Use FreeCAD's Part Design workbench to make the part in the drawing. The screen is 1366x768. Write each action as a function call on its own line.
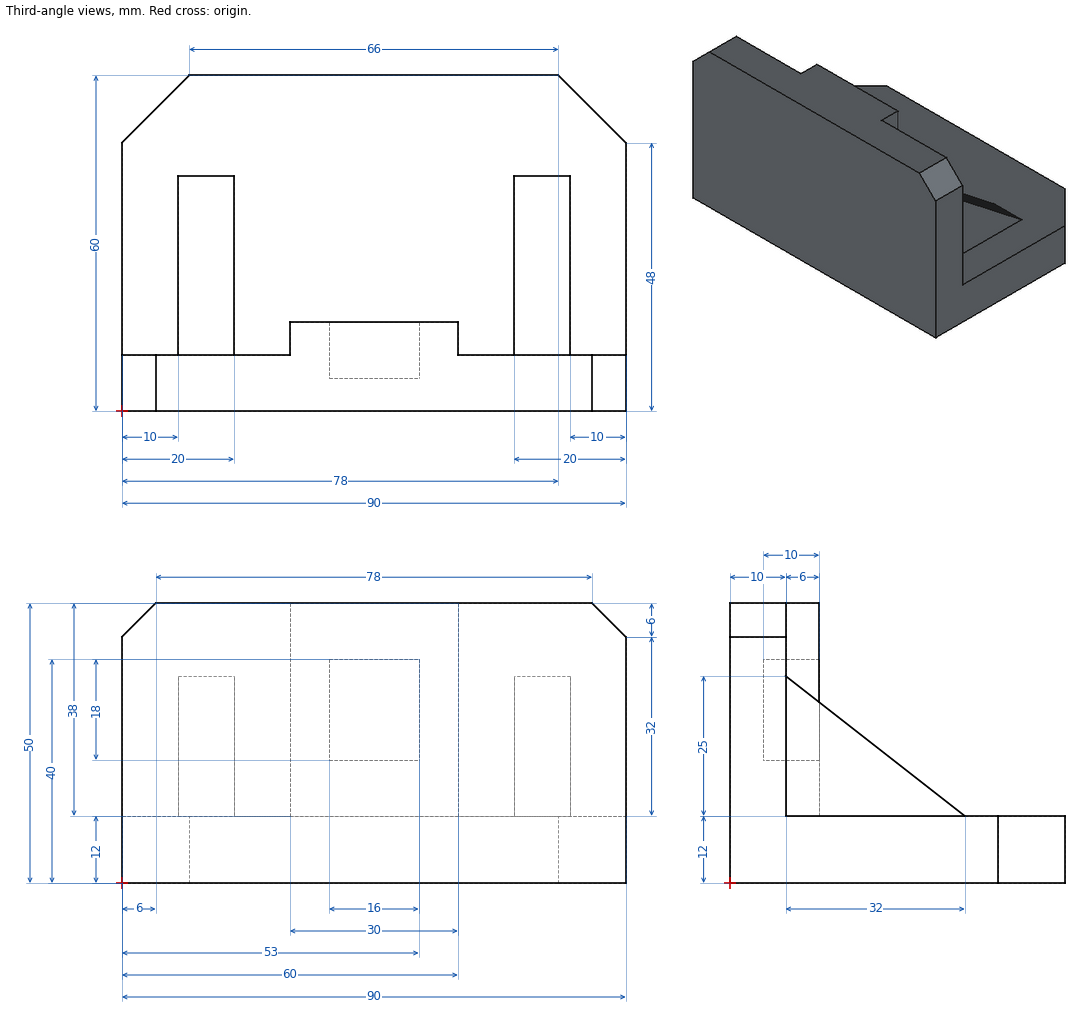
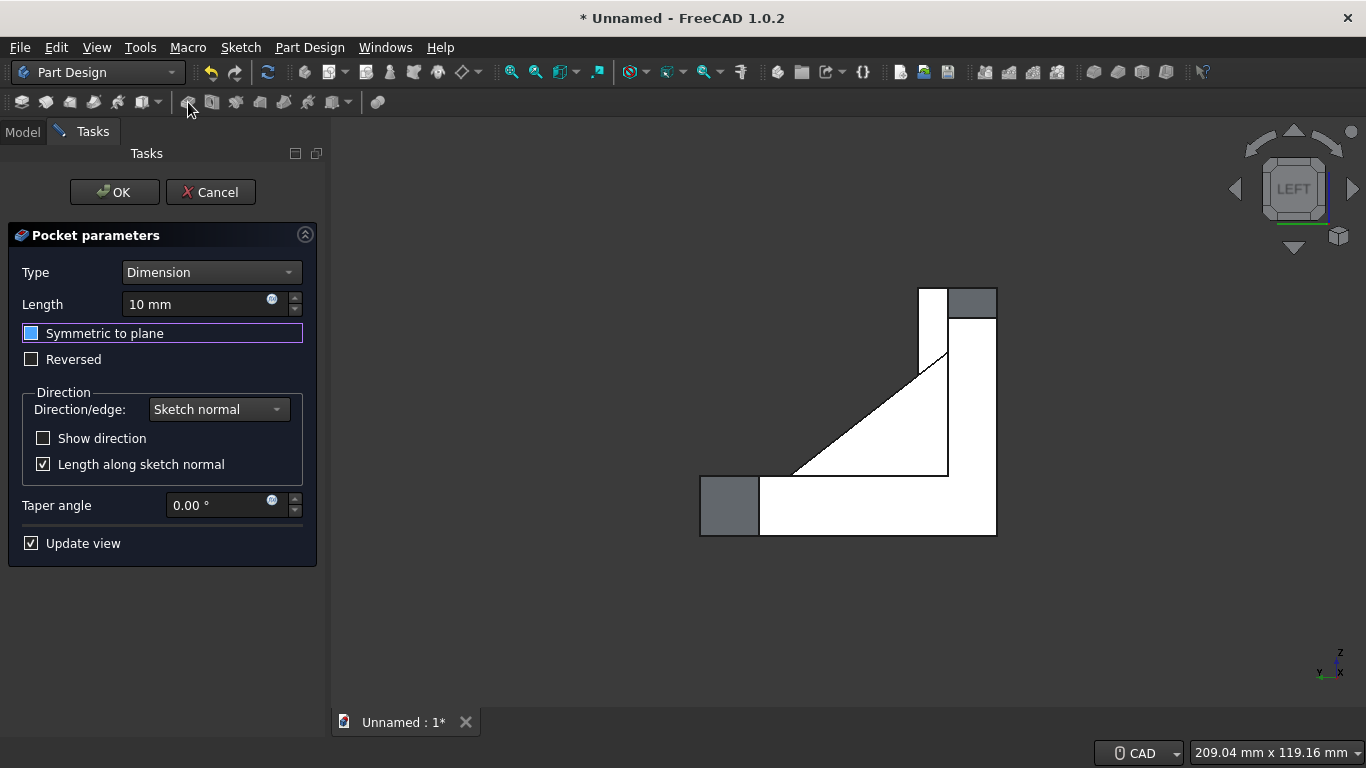
click(115, 192)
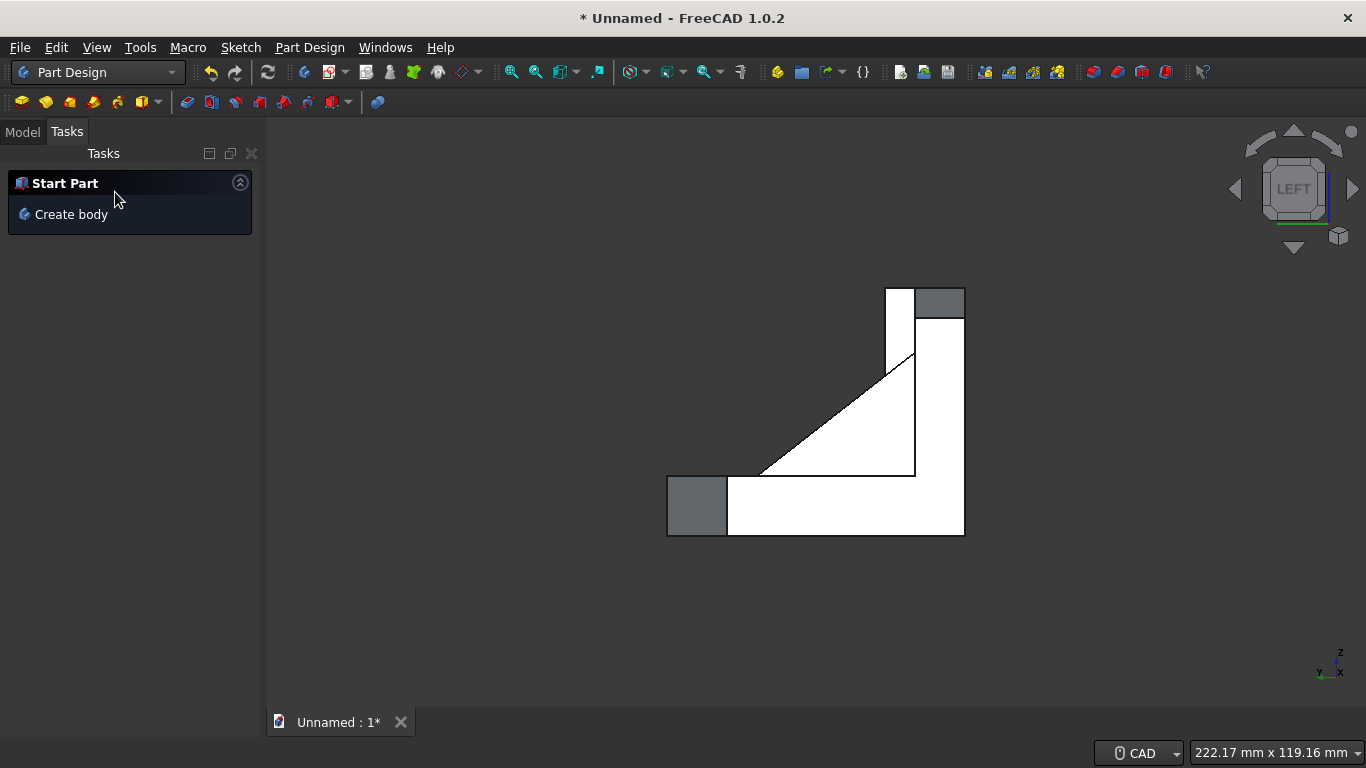
key(0)